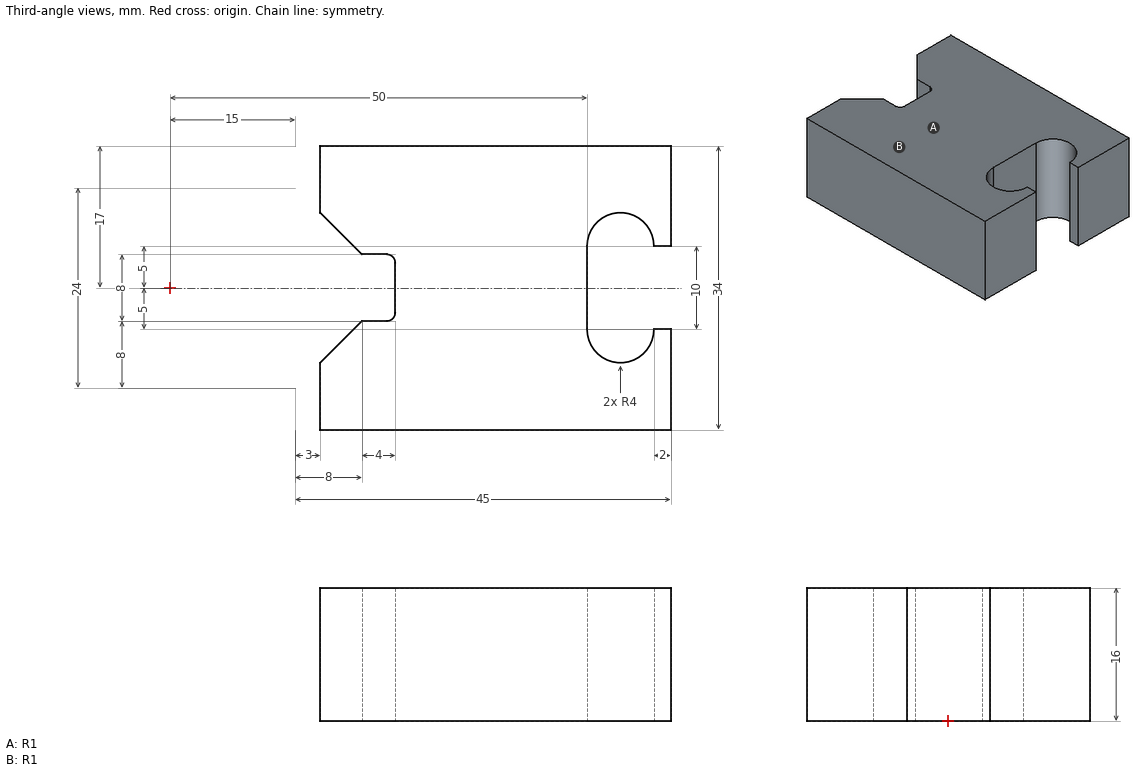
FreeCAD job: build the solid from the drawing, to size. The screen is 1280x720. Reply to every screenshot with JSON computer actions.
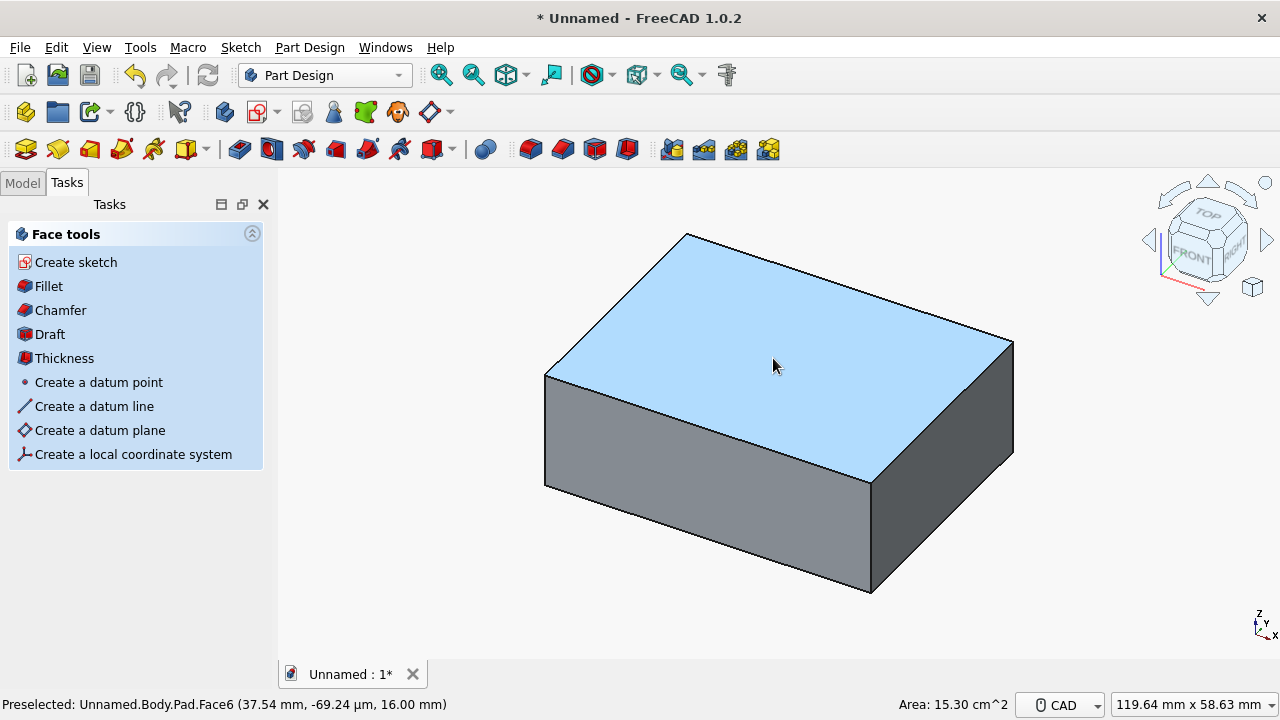
{"action": "left_click", "coordinate": [258, 112]}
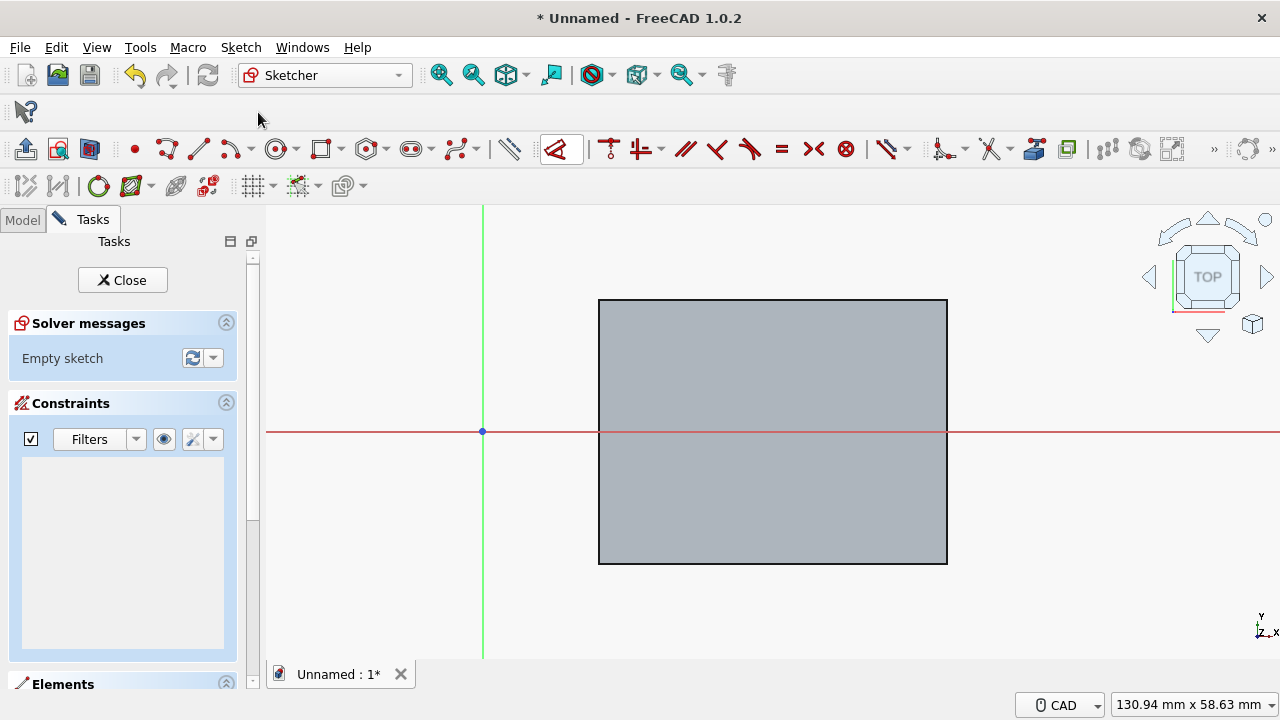
{"action": "scroll", "coordinate": [349, 432], "scroll_direction": "up", "scroll_amount": 2}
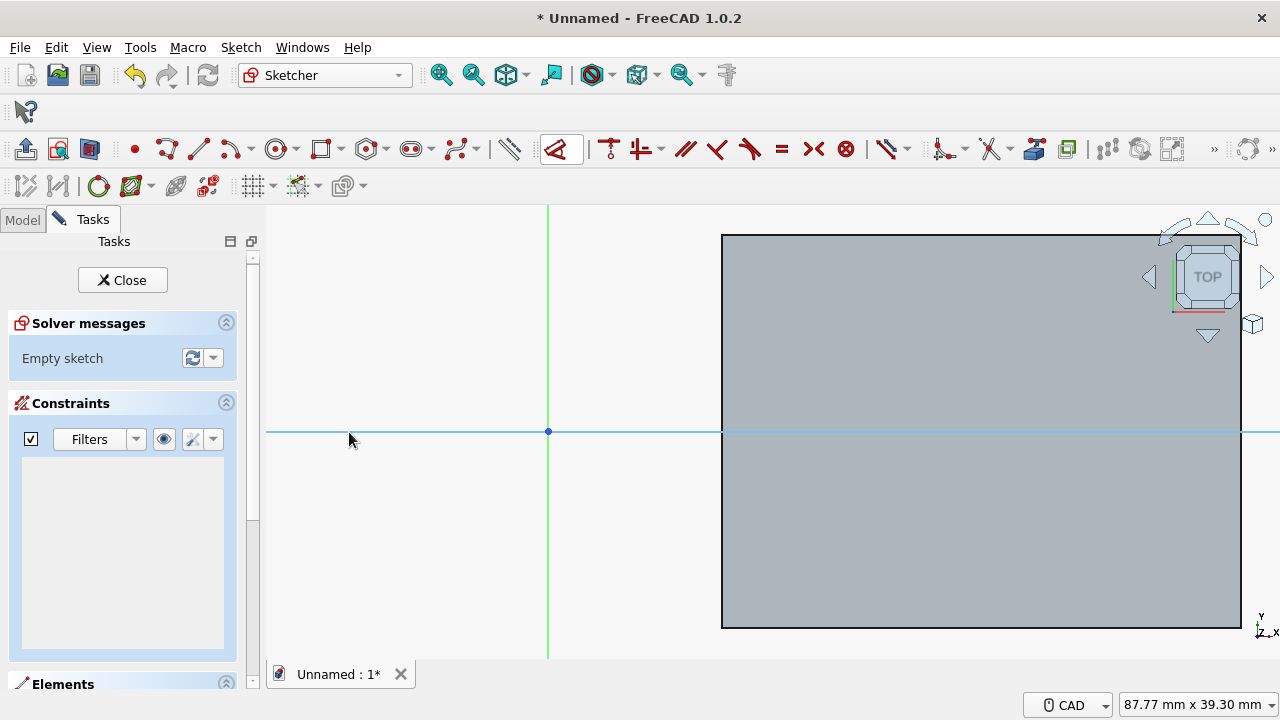
{"action": "left_click", "coordinate": [168, 150]}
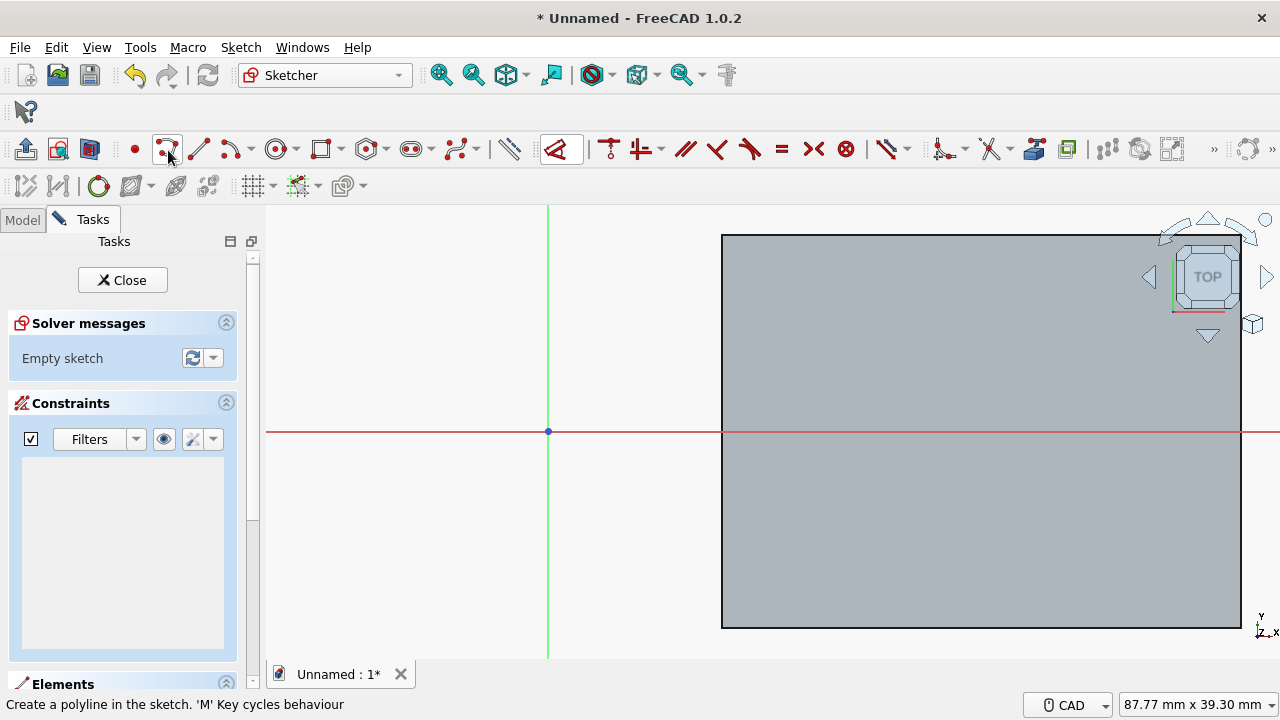
{"action": "left_click", "coordinate": [722, 293]}
{"action": "left_click", "coordinate": [722, 570]}
{"action": "left_click", "coordinate": [814, 478]}
{"action": "left_click", "coordinate": [860, 478]}
{"action": "left_click", "coordinate": [860, 386]}
{"action": "left_click", "coordinate": [814, 386]}
{"action": "left_click", "coordinate": [722, 294]}
{"action": "key", "text": "Escape"}
{"action": "key", "text": "Escape"}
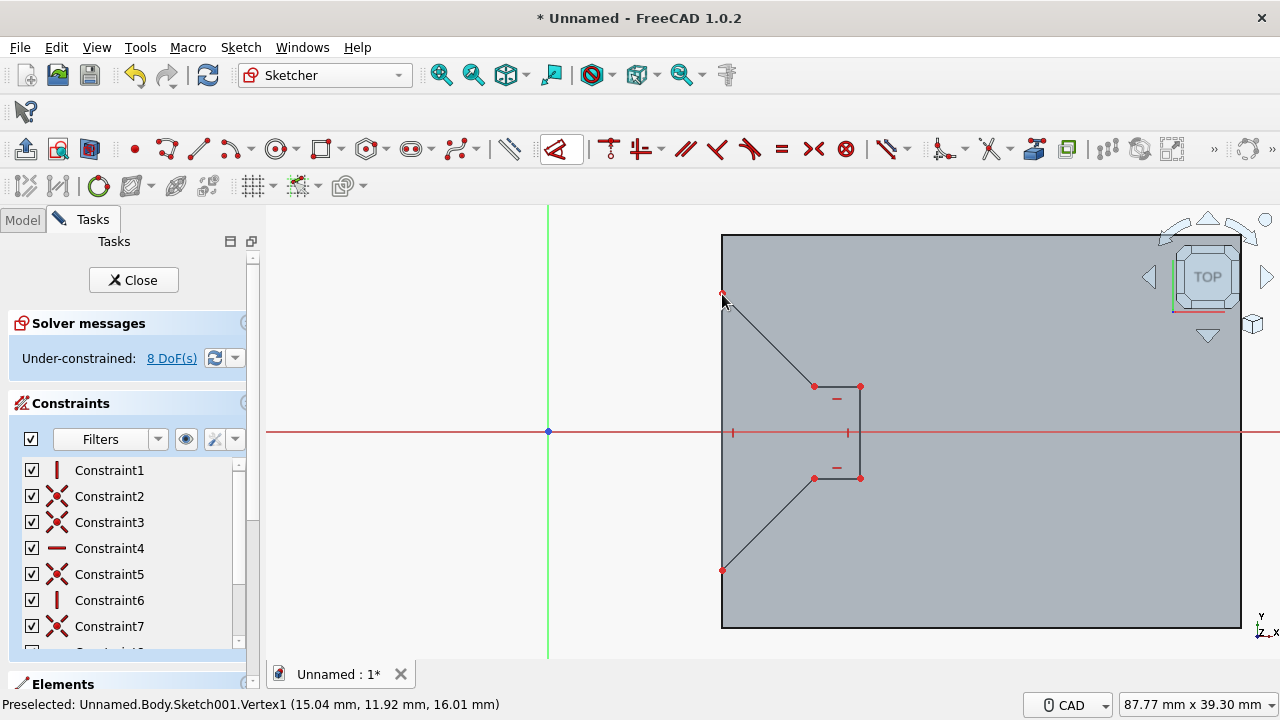
{"action": "left_click", "coordinate": [814, 479]}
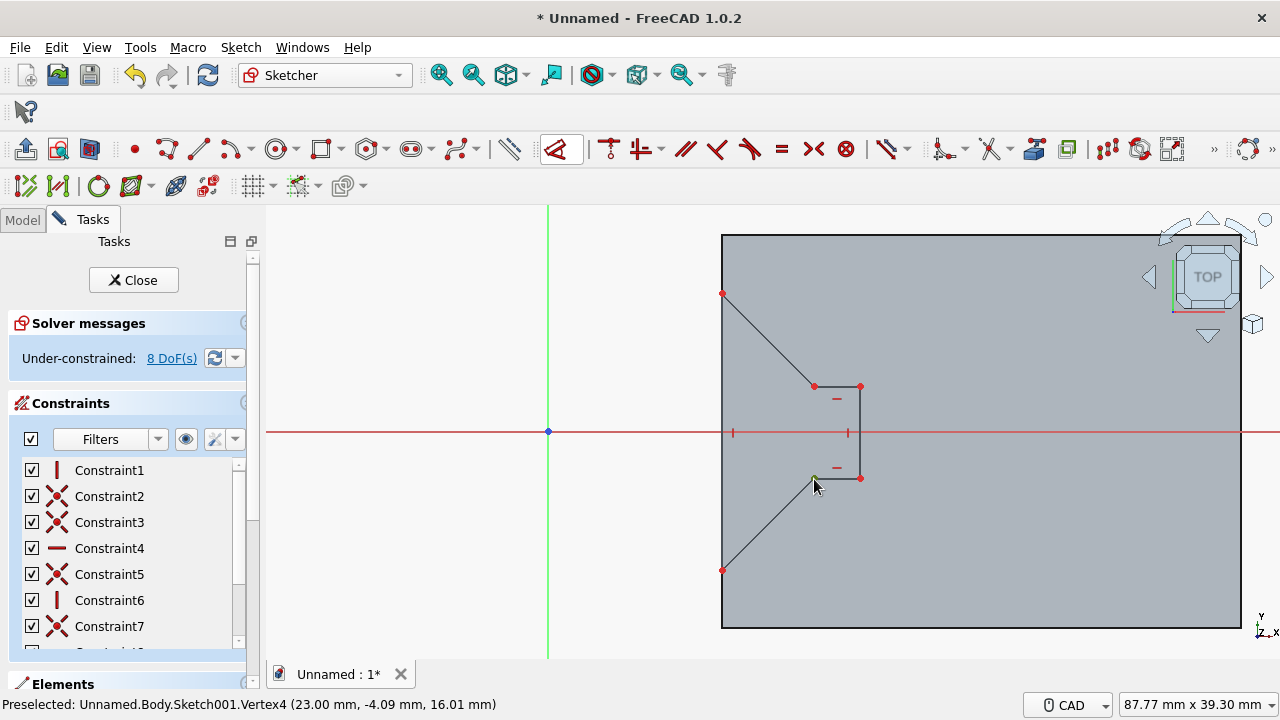
{"action": "left_click", "coordinate": [814, 387]}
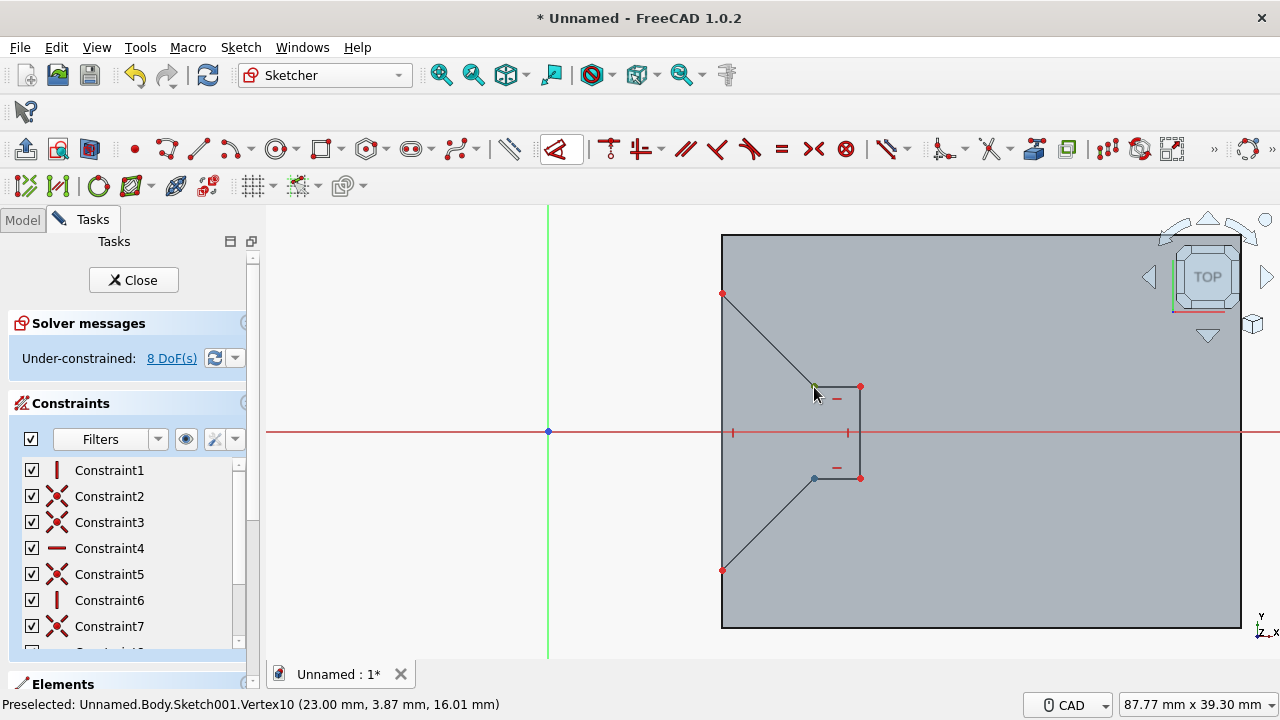
{"action": "left_click", "coordinate": [353, 432]}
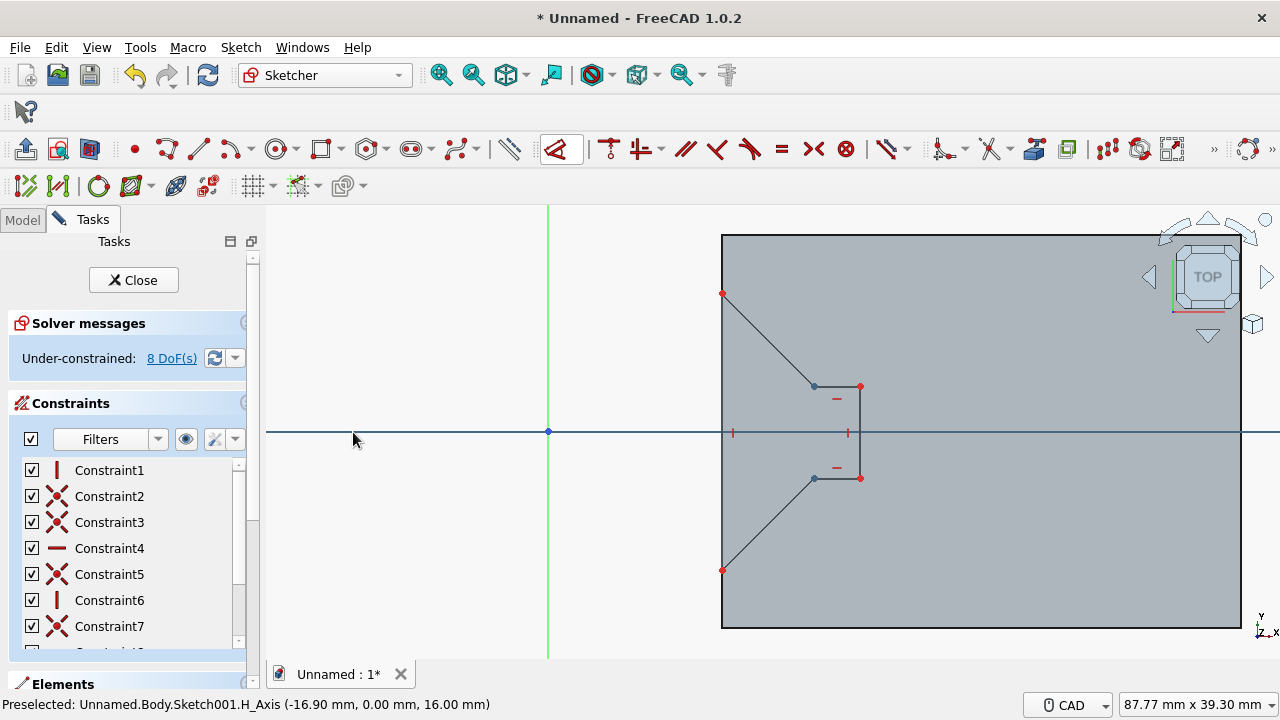
{"action": "left_click", "coordinate": [814, 150]}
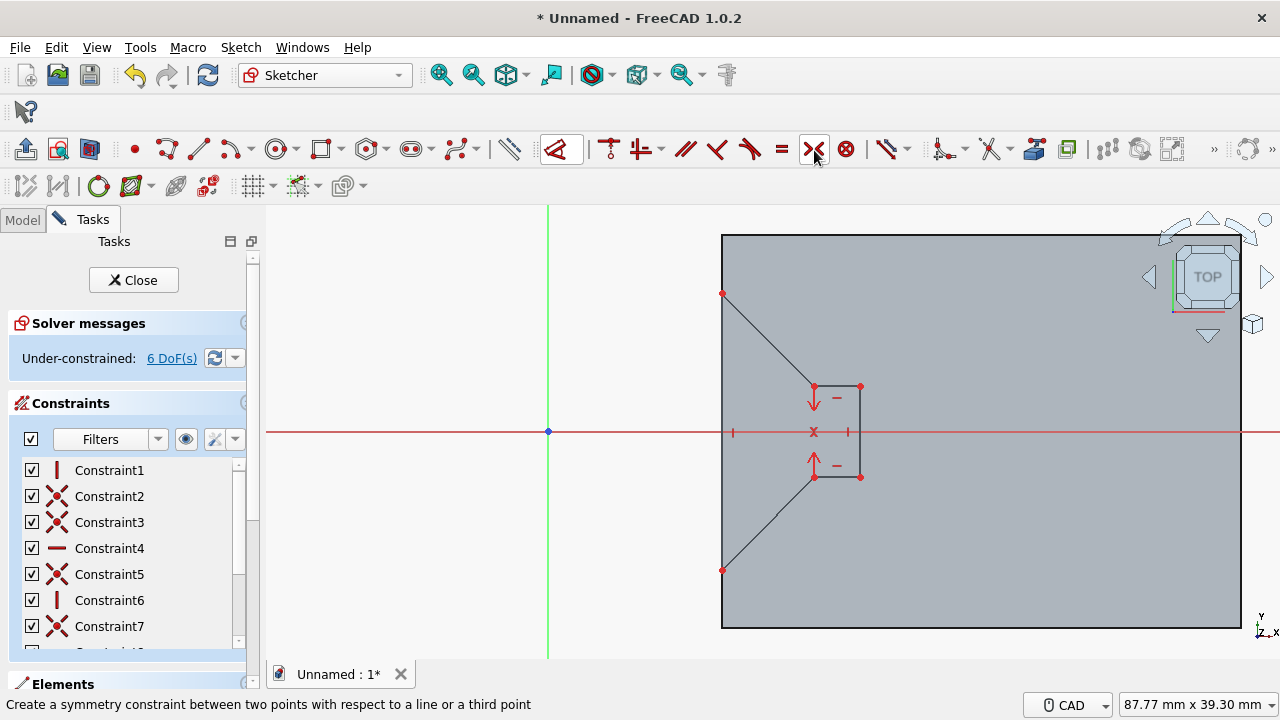
{"action": "left_click", "coordinate": [828, 477]}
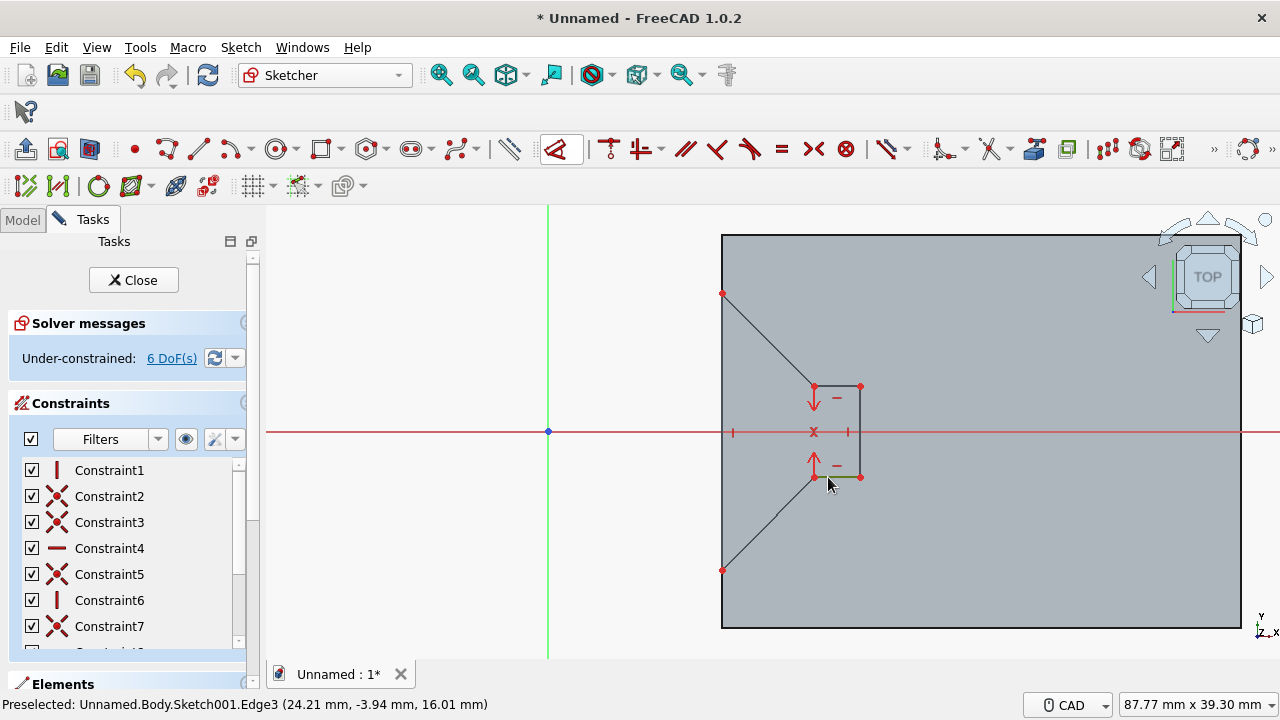
{"action": "key", "text": "l"}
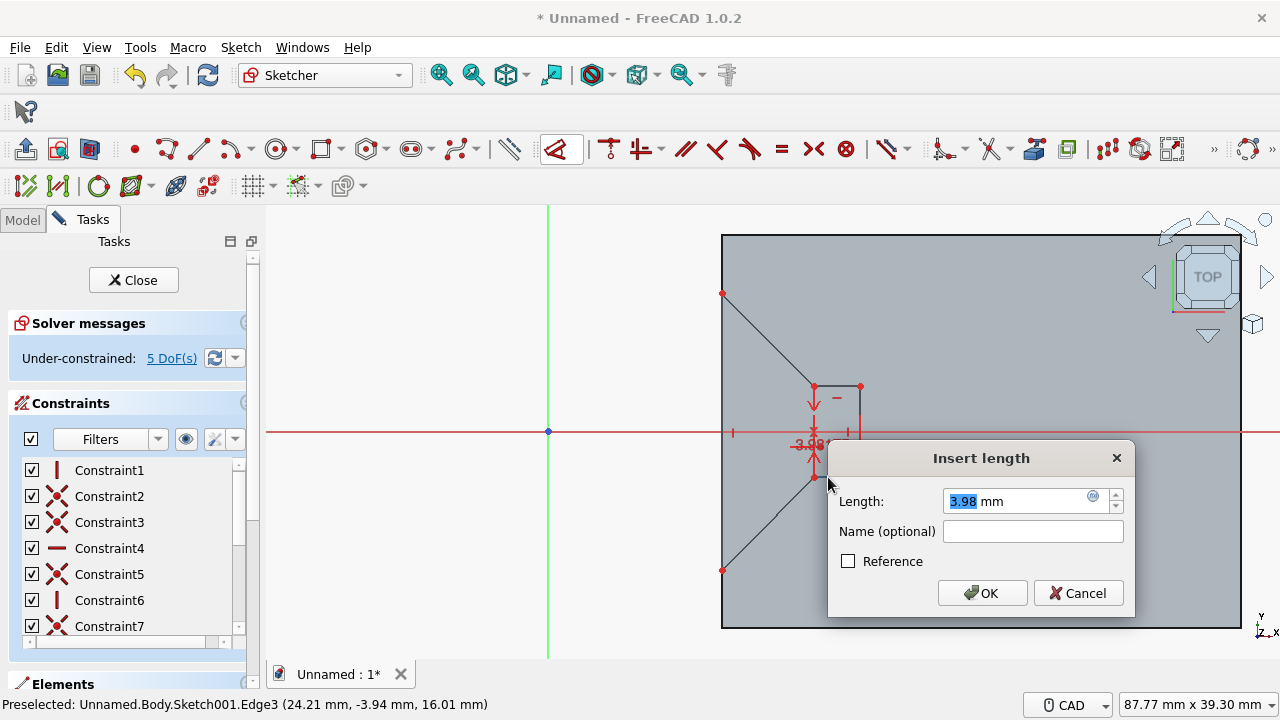
{"action": "type", "text": "4"}
{"action": "key", "text": "Return"}